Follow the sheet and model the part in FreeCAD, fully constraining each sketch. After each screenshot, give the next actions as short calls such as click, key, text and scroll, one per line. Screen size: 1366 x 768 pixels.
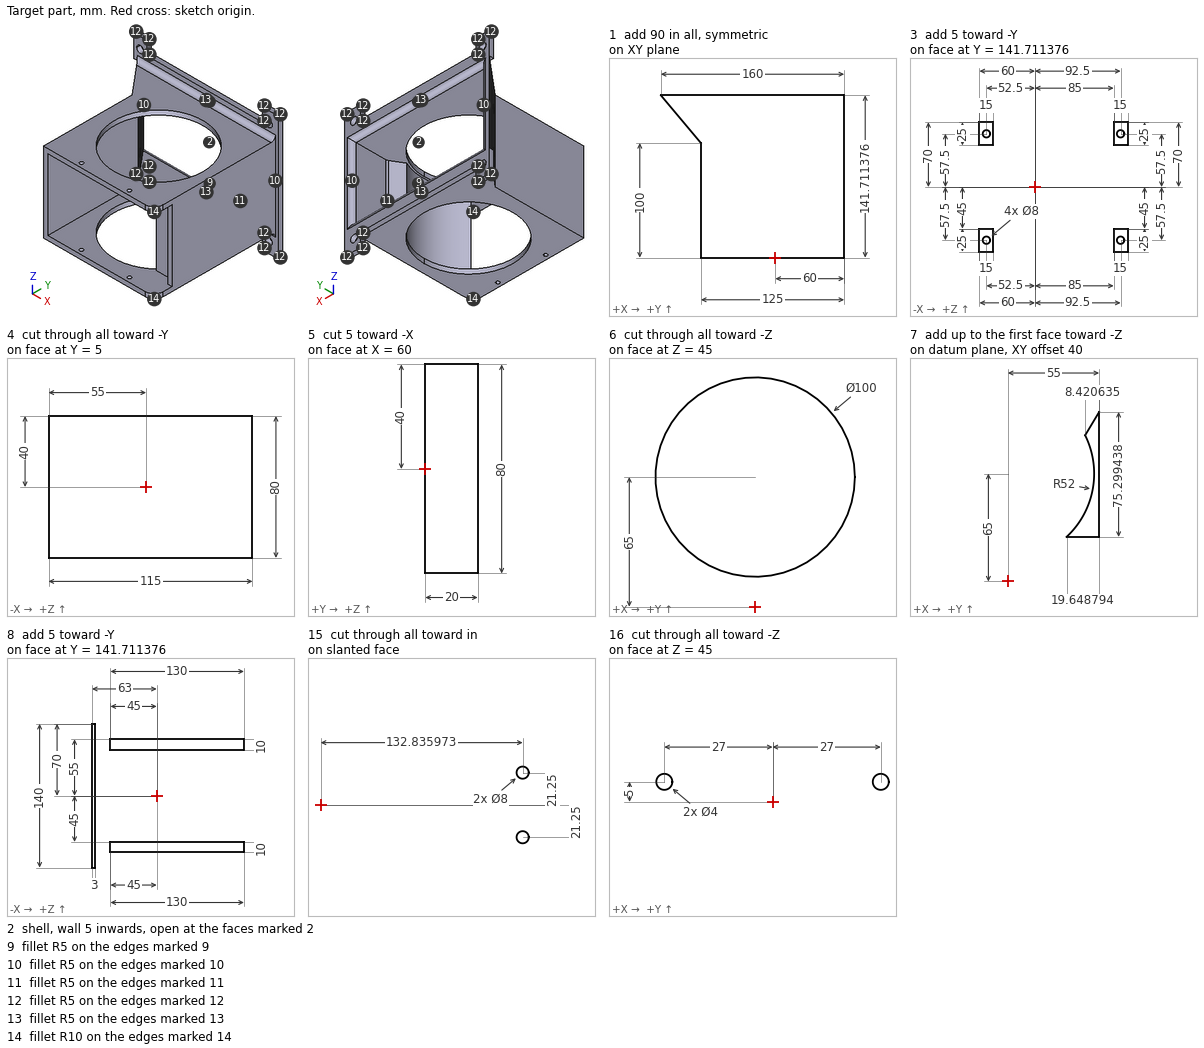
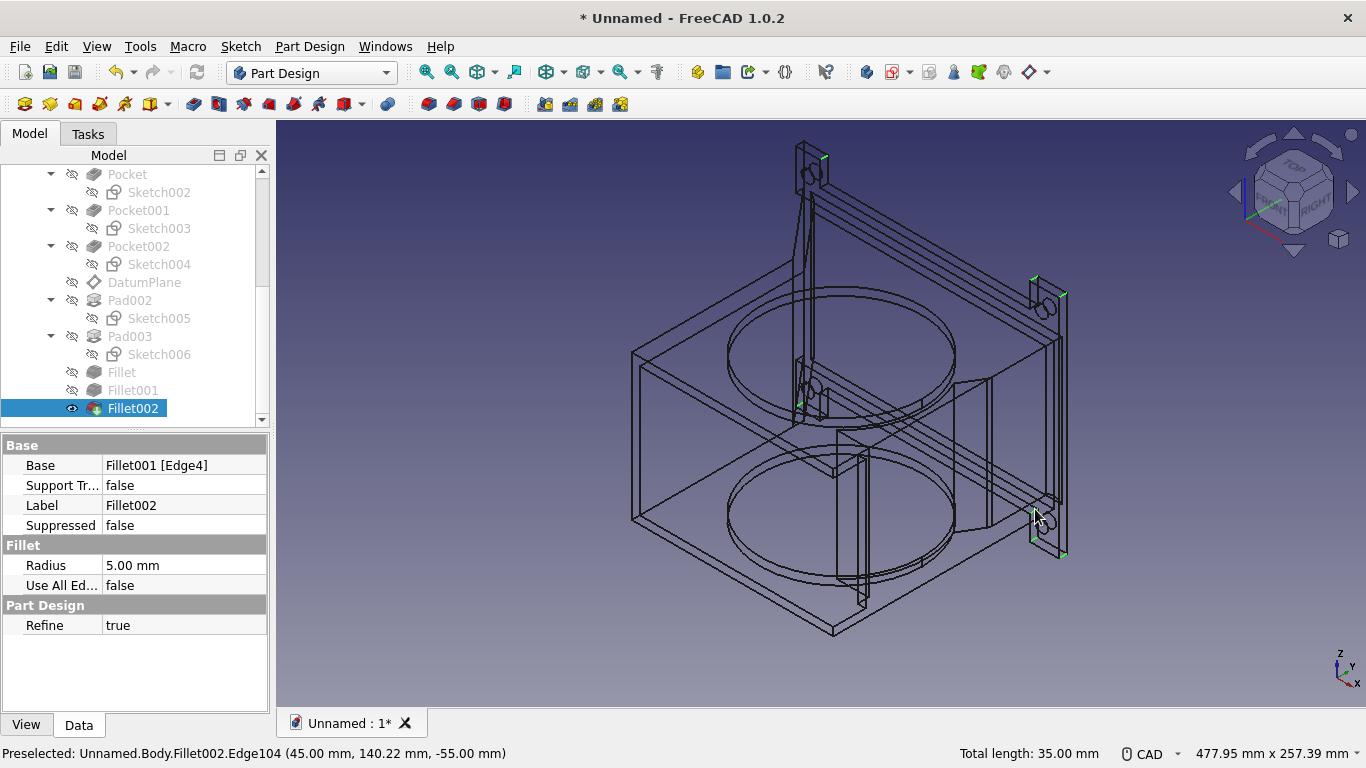
click(827, 388, ctrl)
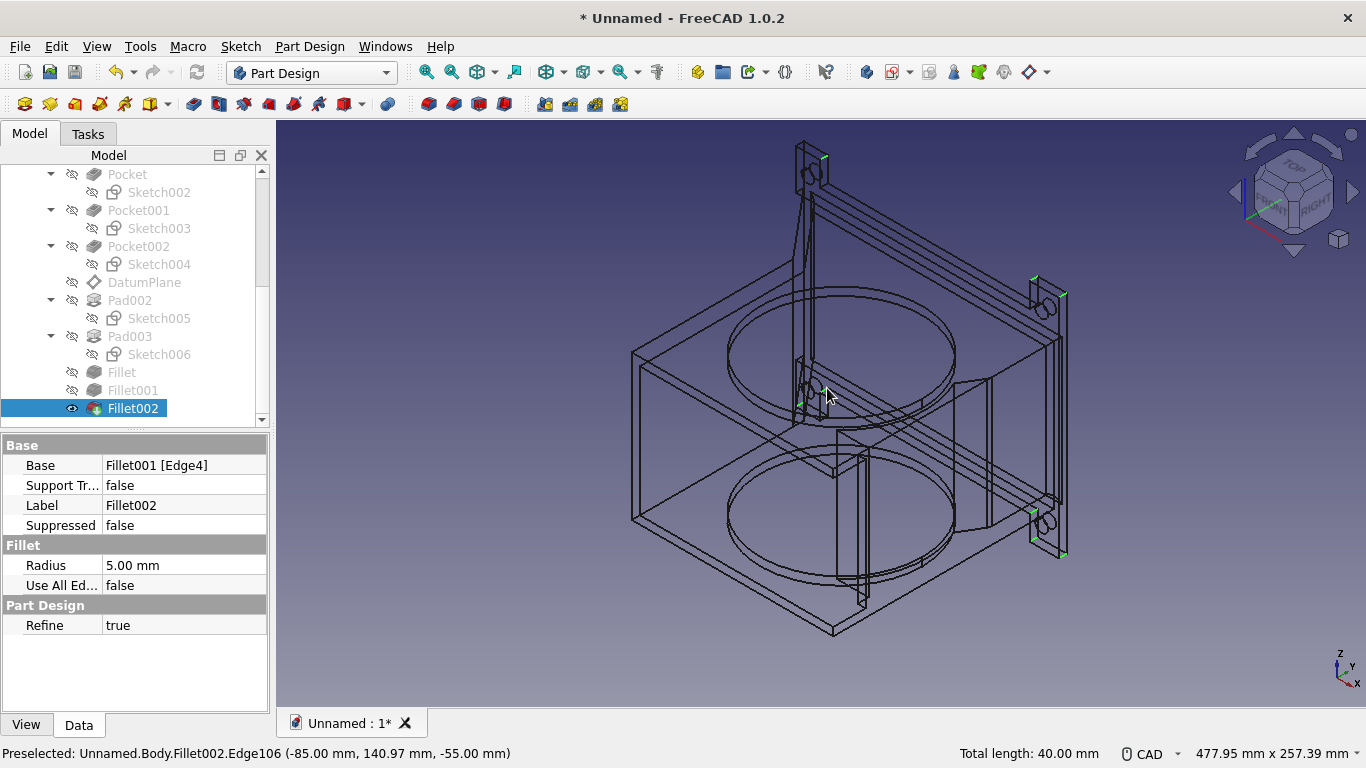
scroll(1034, 306, up, 7)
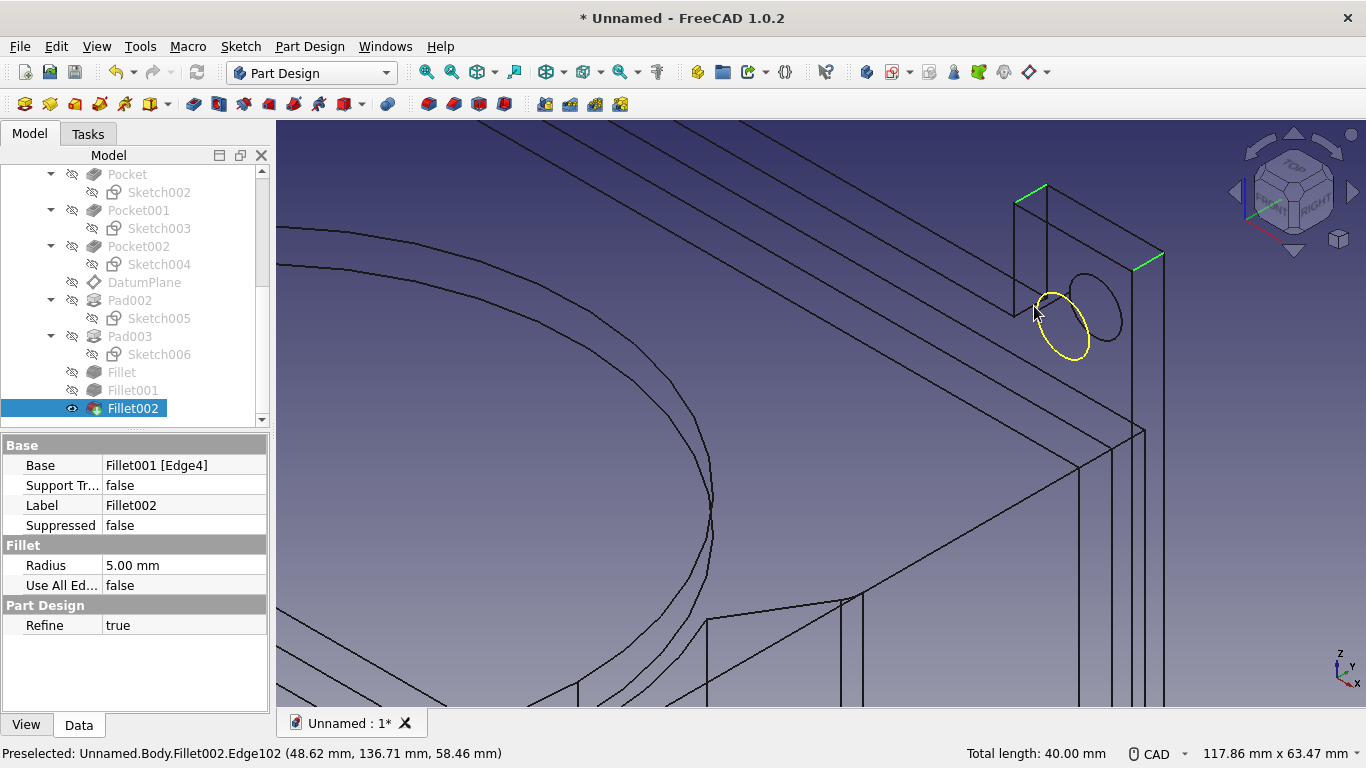
click(1030, 306, ctrl)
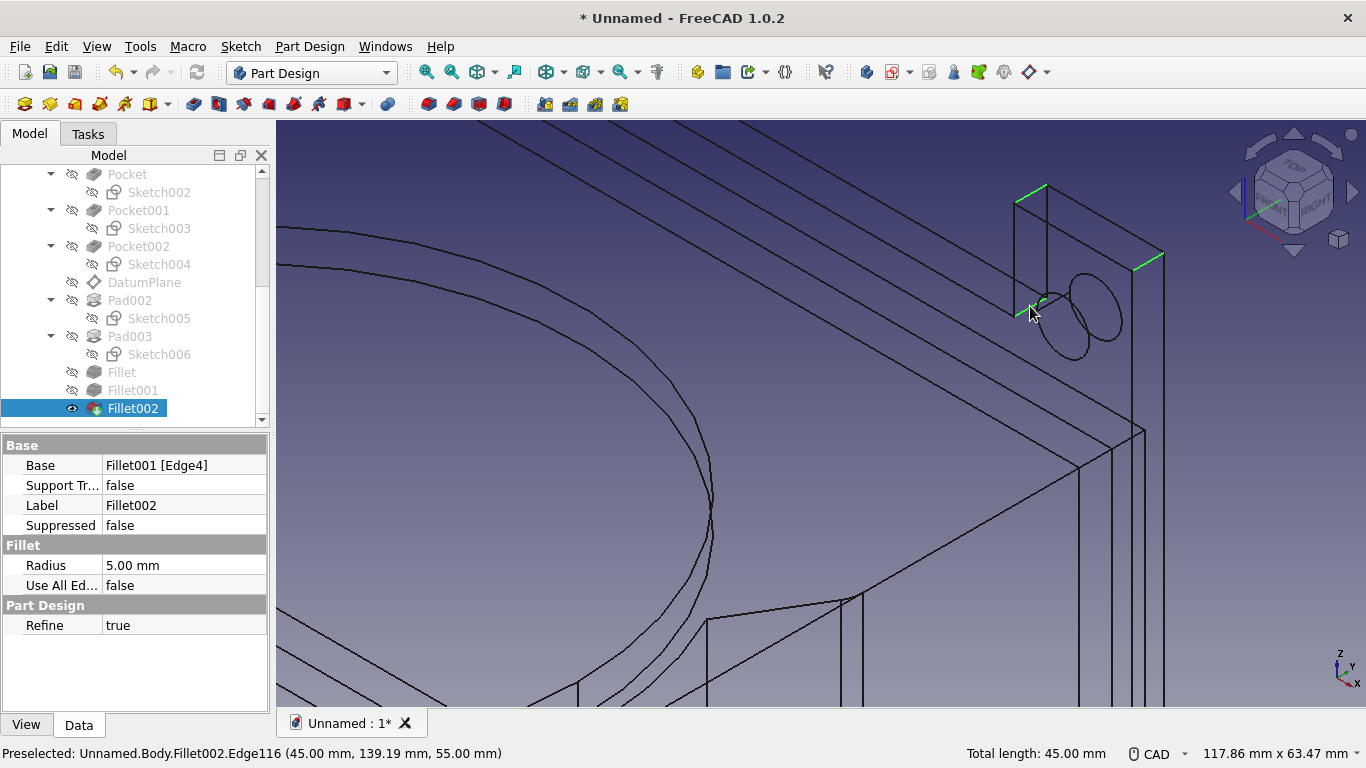
key(v)
key(f)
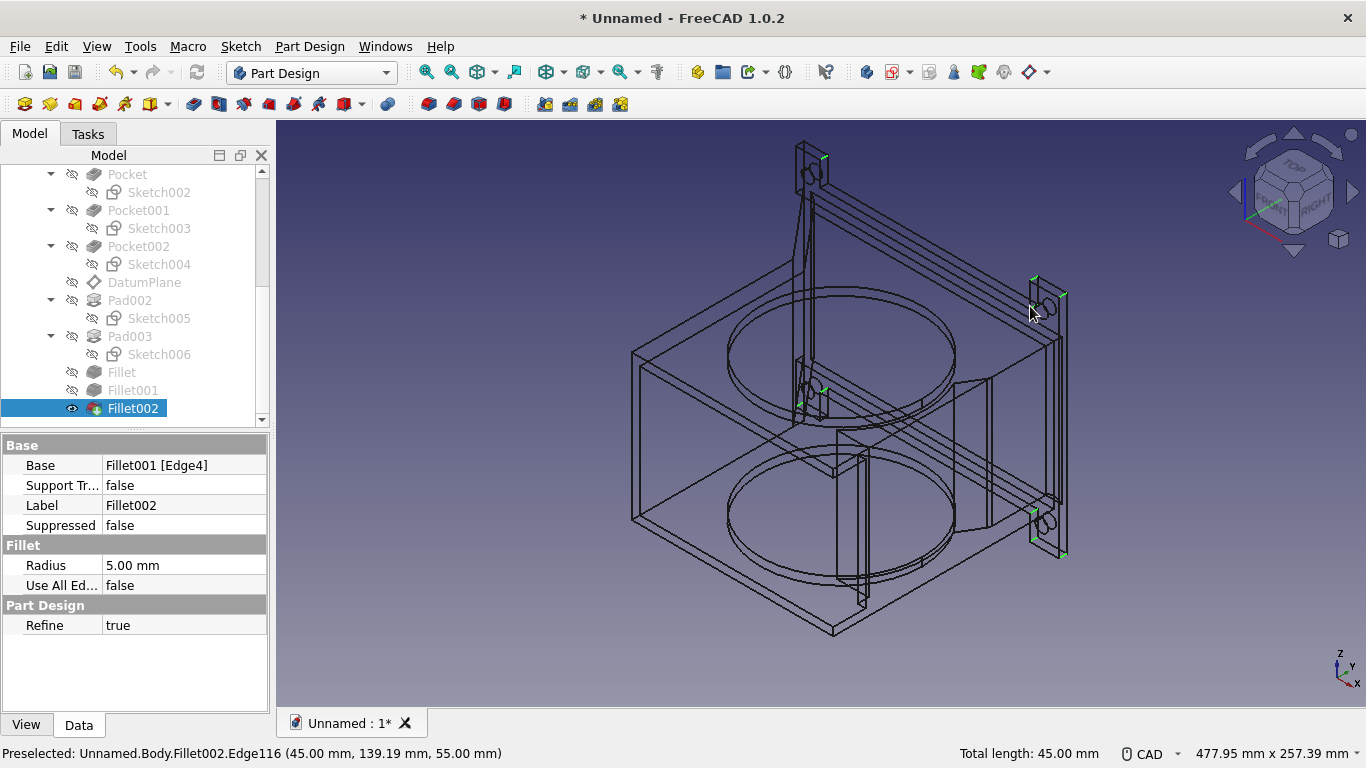
key(2)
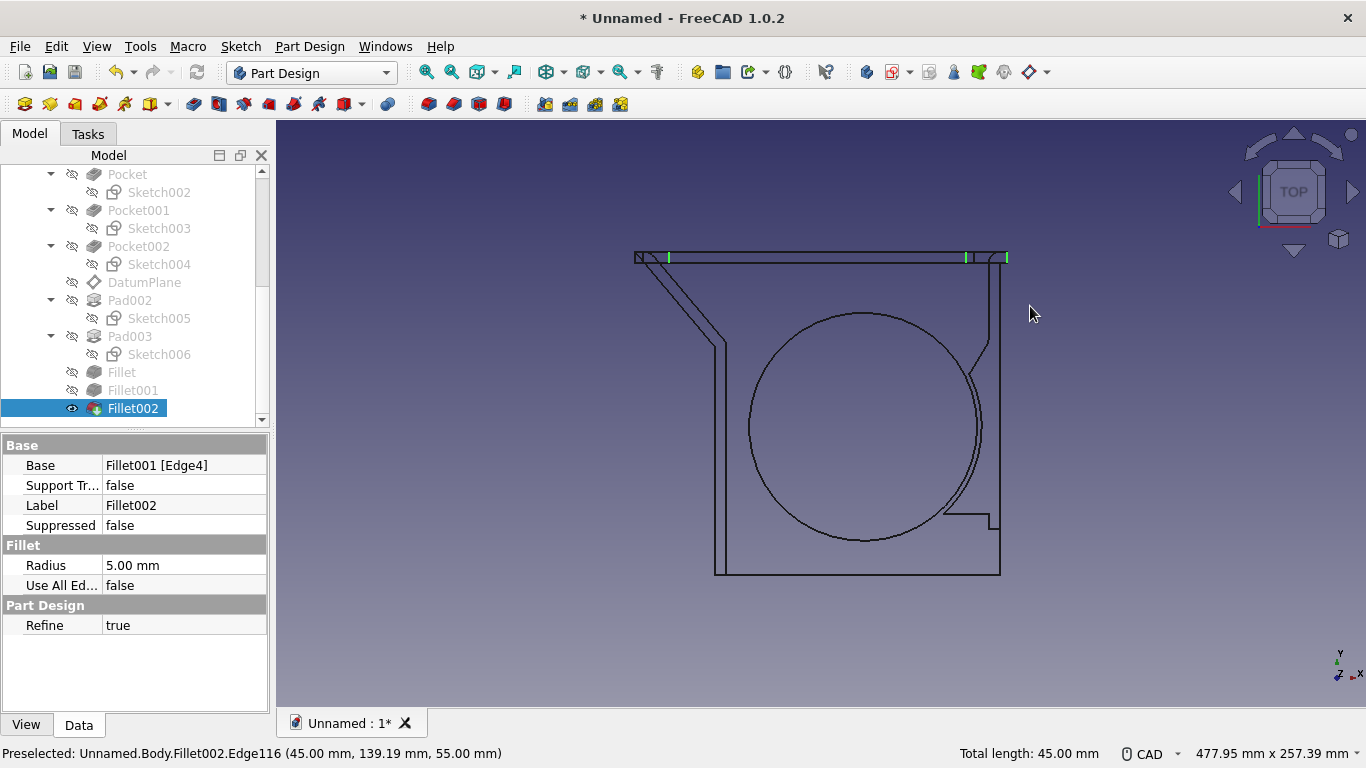
scroll(669, 257, up, 7)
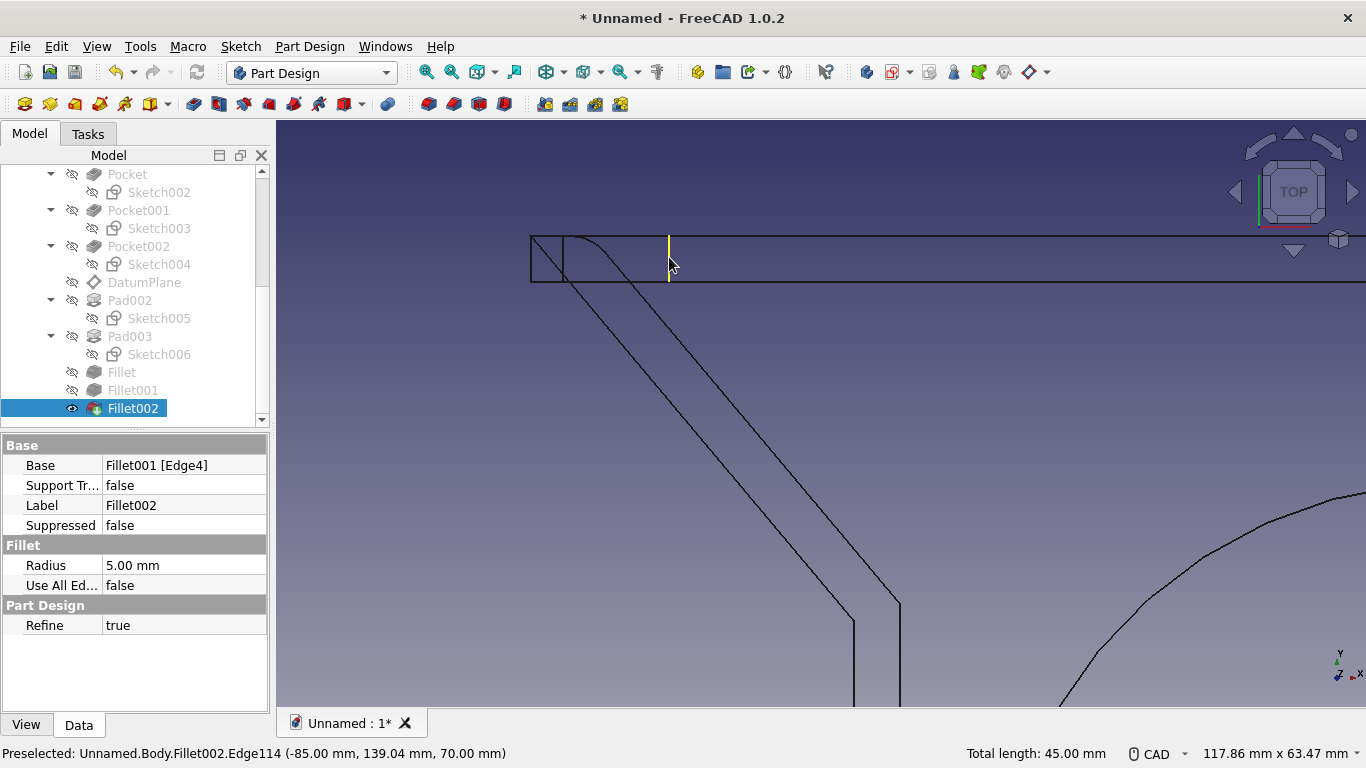
click(531, 258, ctrl)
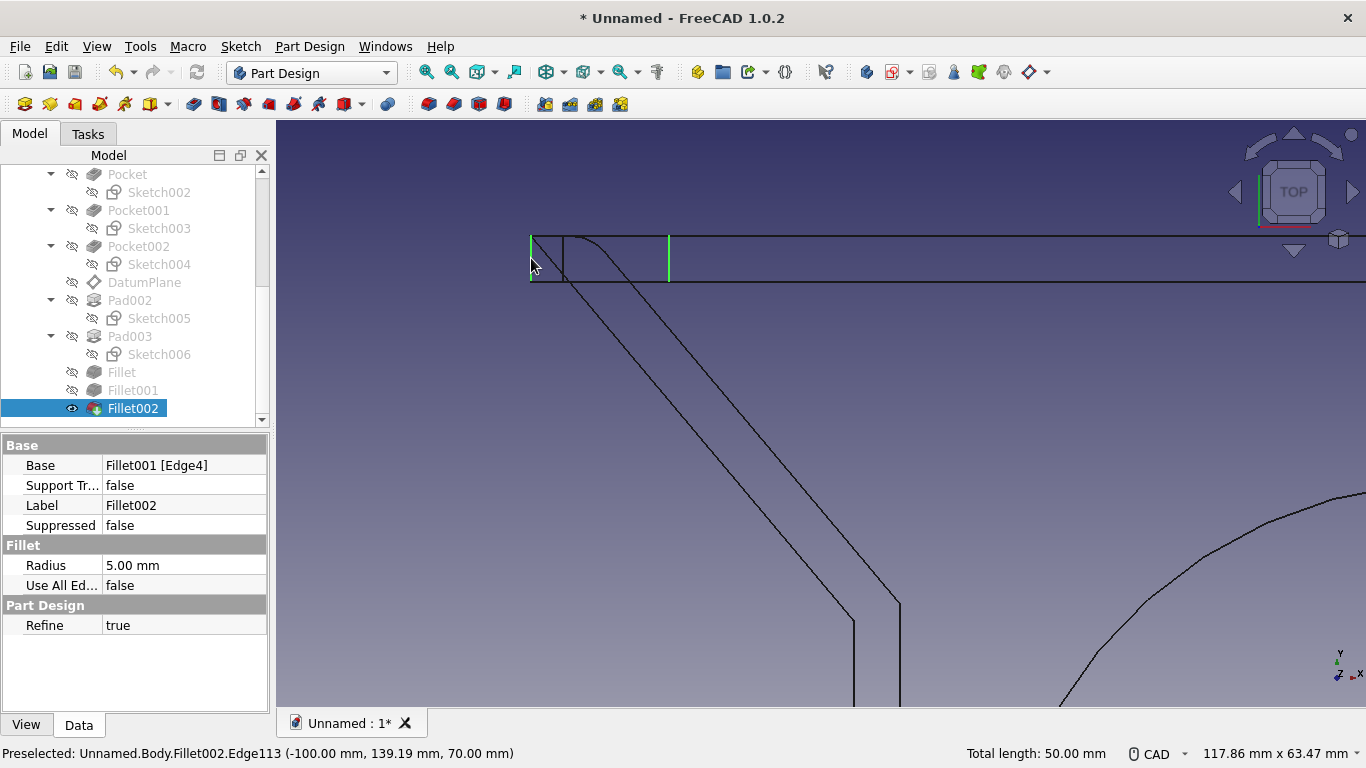
key(v)
key(f)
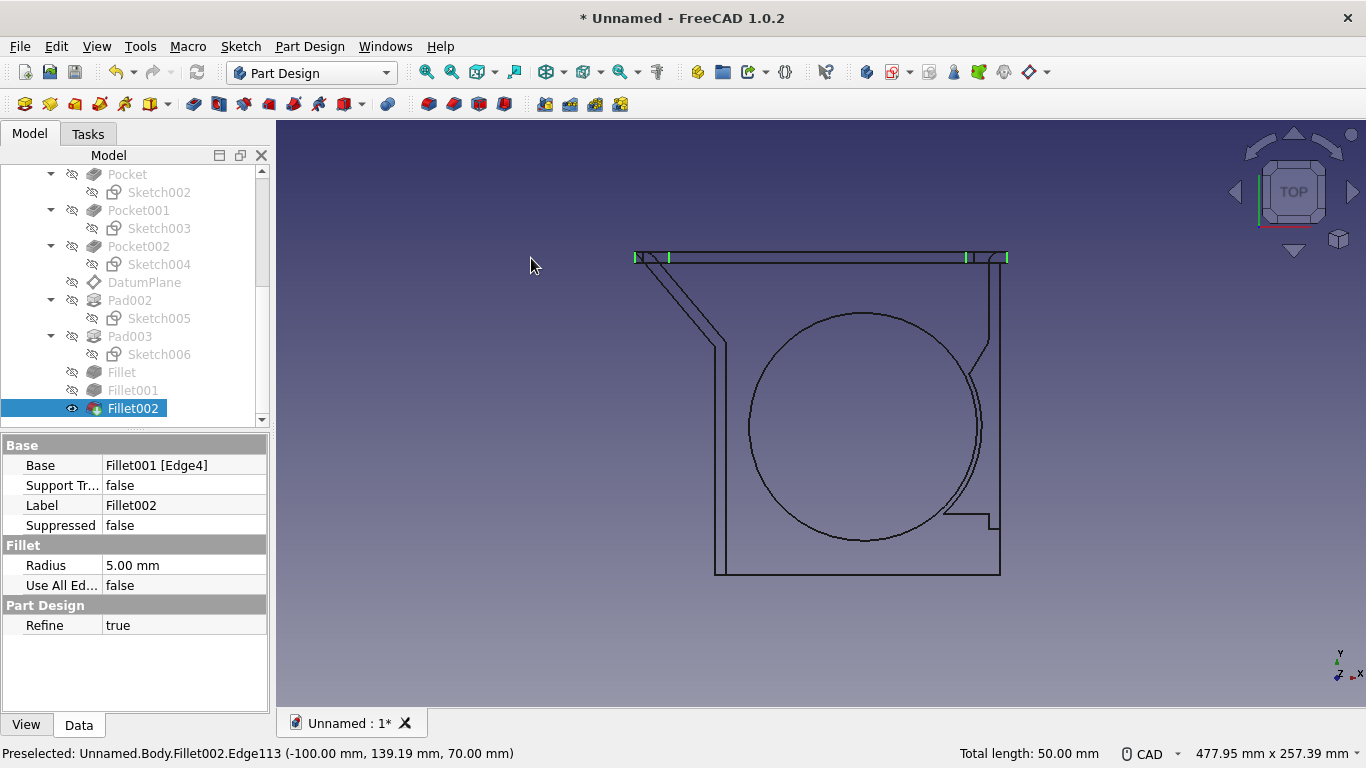
key(1)